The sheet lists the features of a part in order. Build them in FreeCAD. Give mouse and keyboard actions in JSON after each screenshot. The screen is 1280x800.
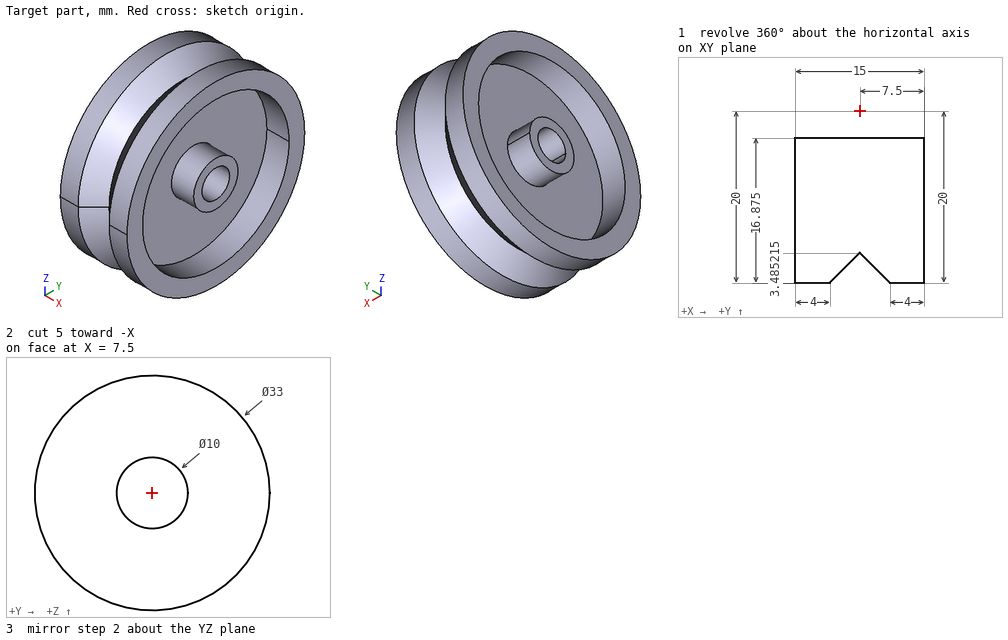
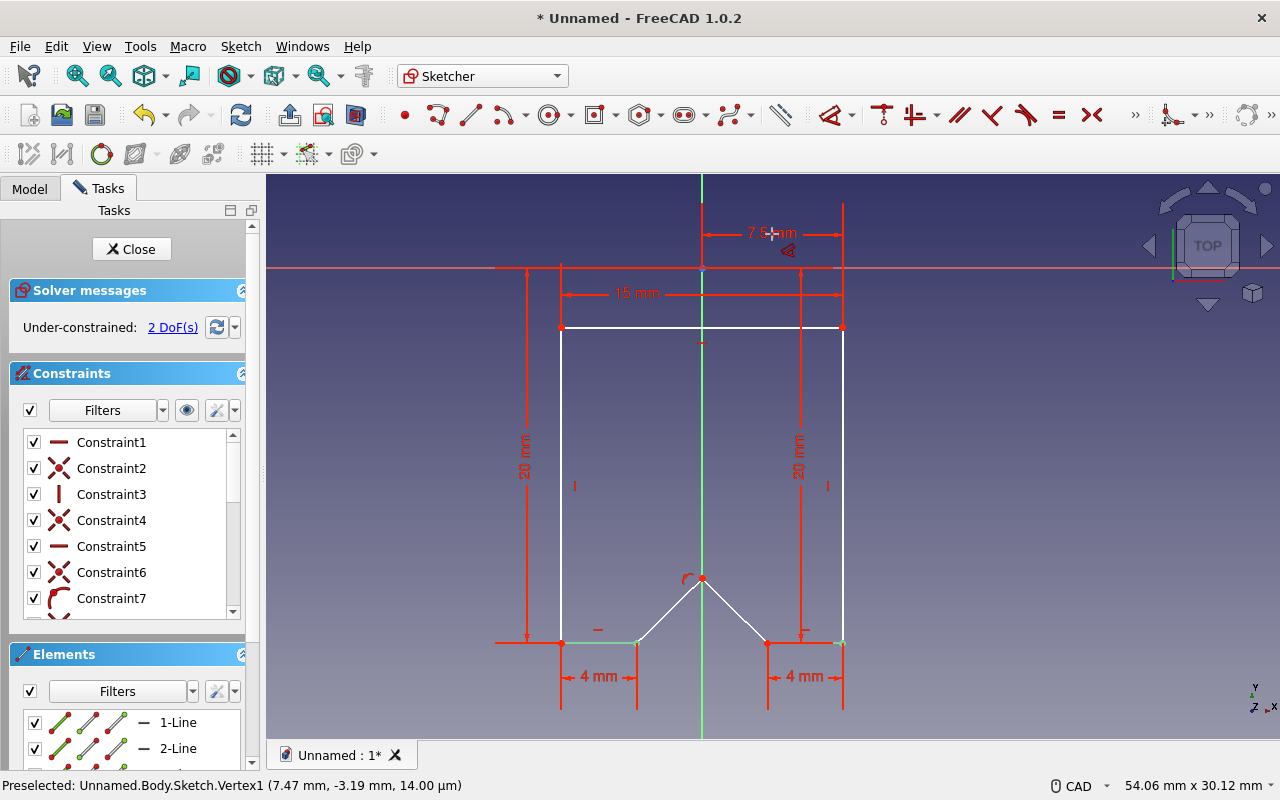
{"action": "left_click", "coordinate": [561, 423]}
{"action": "left_click", "coordinate": [527, 486]}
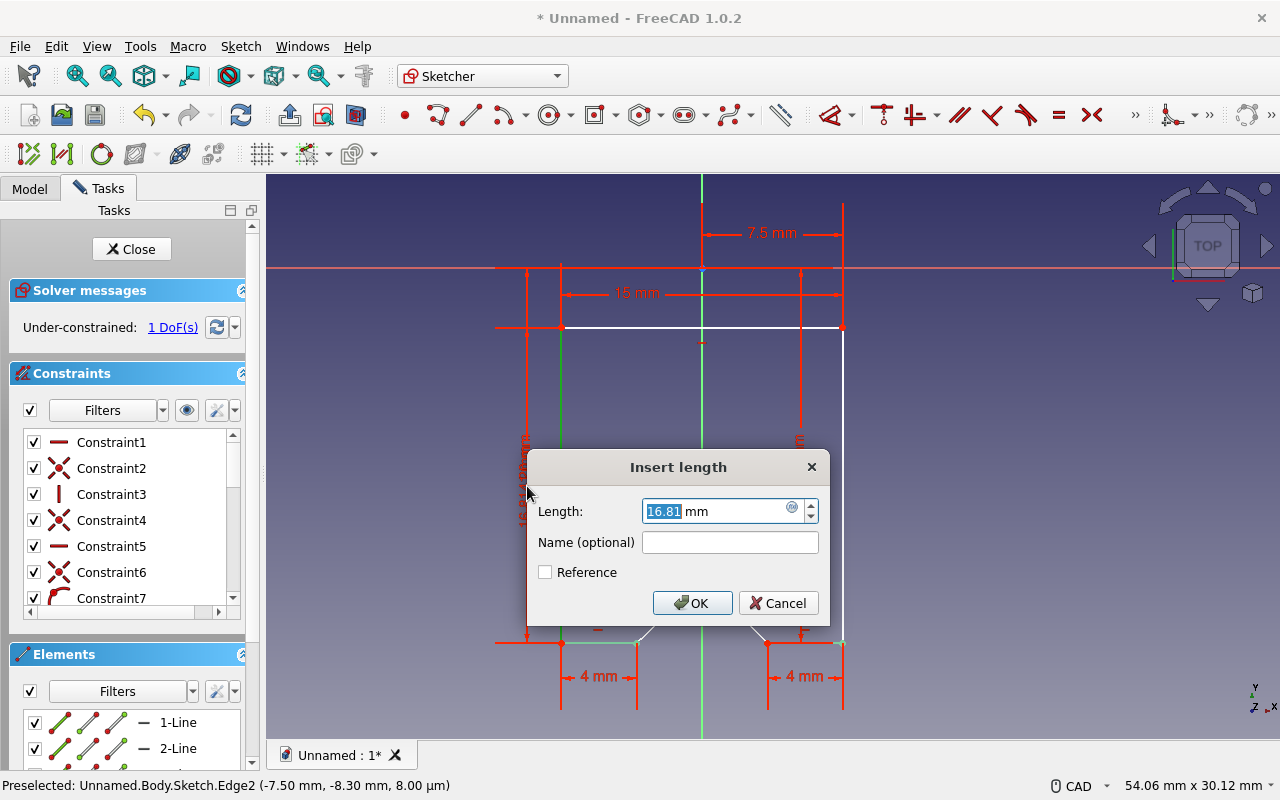
{"action": "type", "text": "16.875"}
{"action": "key", "text": "Return"}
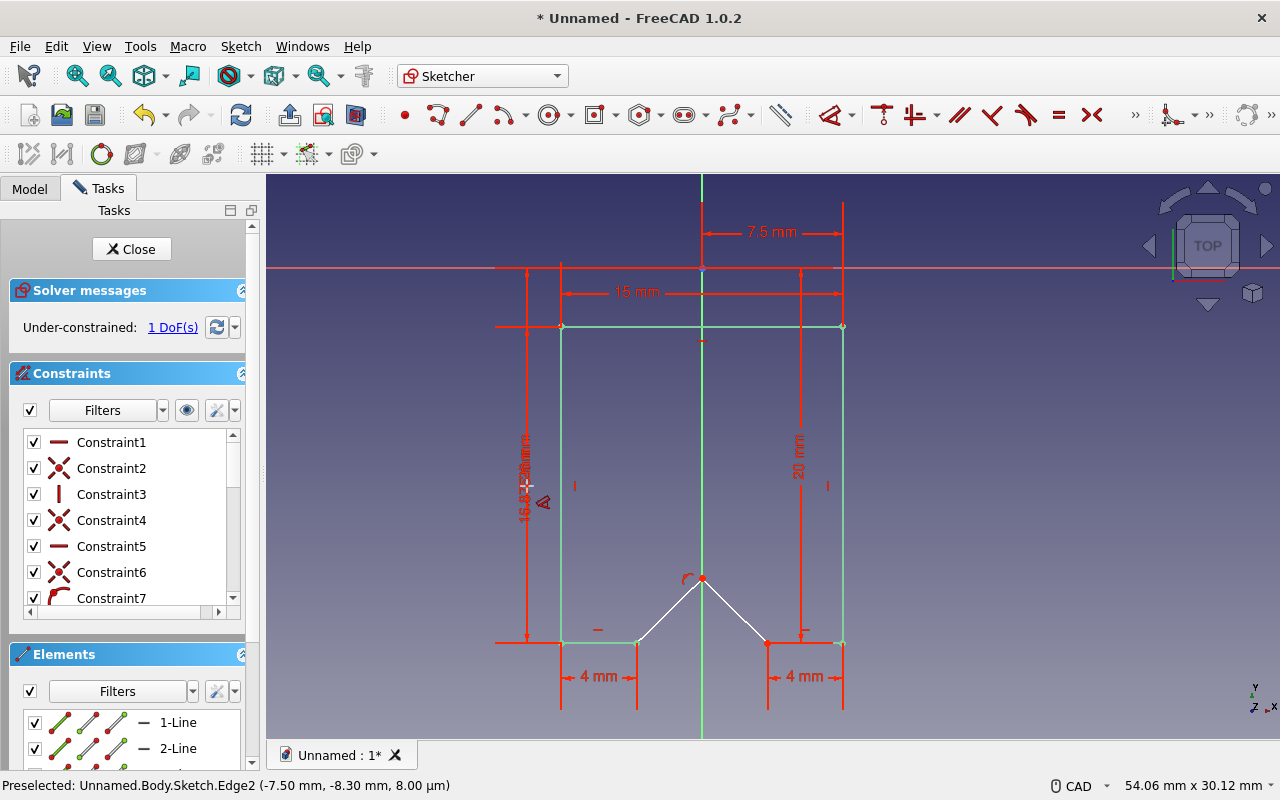
{"action": "left_click", "coordinate": [656, 624]}
{"action": "left_click", "coordinate": [603, 611]}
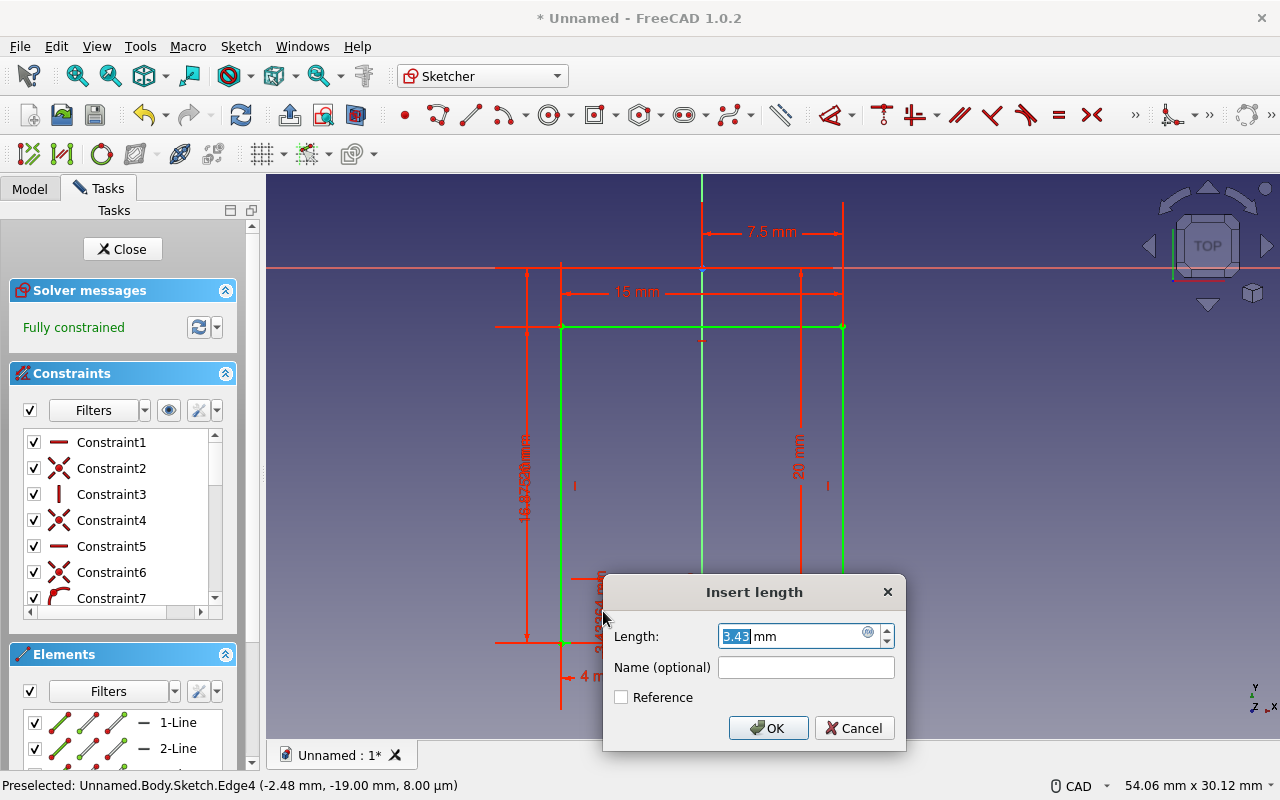
{"action": "type", "text": "3.485215"}
{"action": "key", "text": "Return"}
{"action": "key", "text": "Escape"}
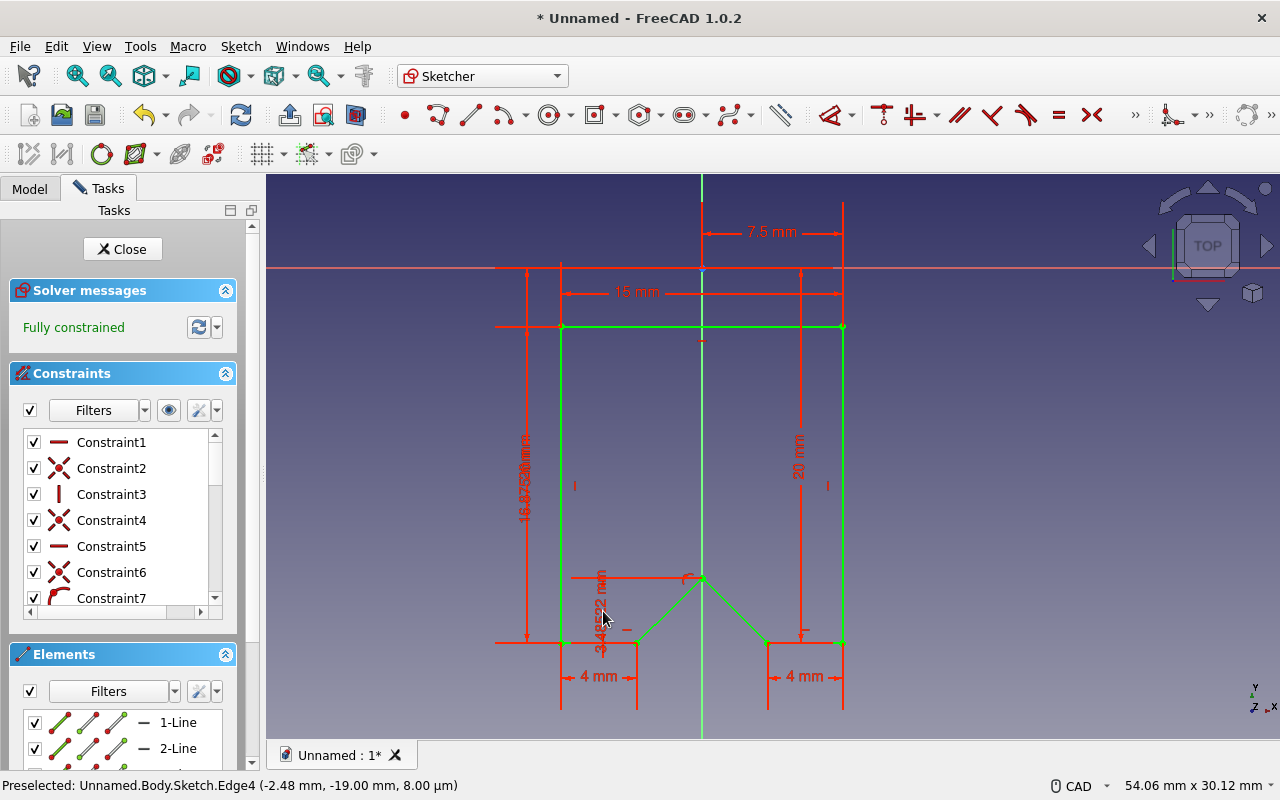
{"action": "left_click", "coordinate": [123, 249]}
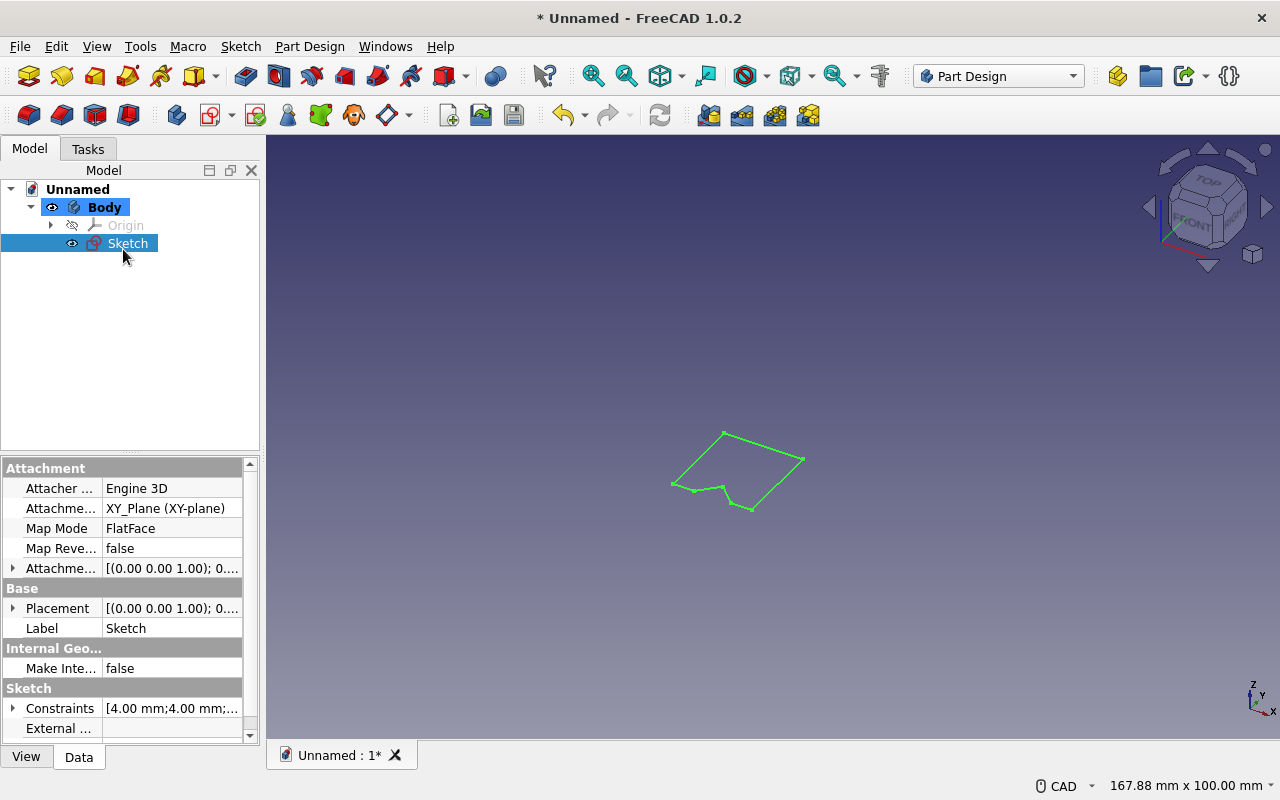
{"action": "left_click", "coordinate": [62, 76]}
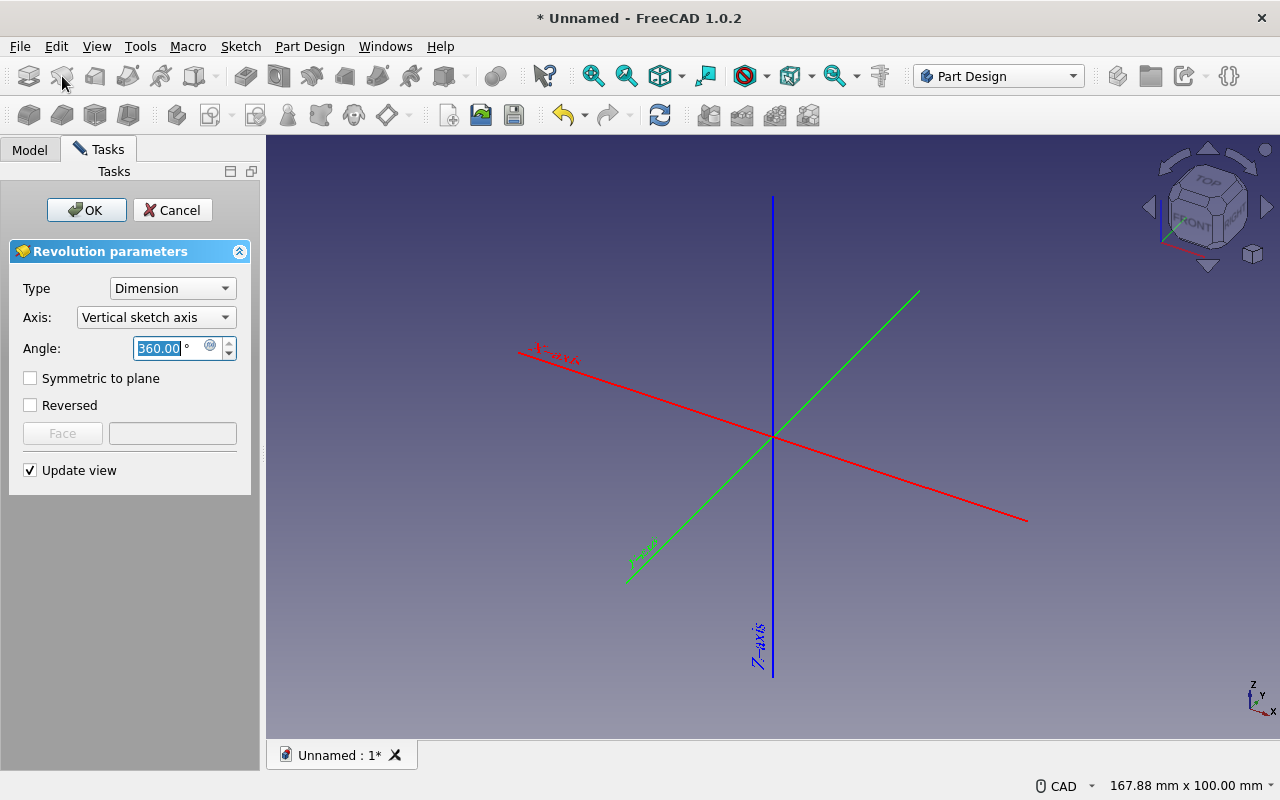
{"action": "left_click", "coordinate": [157, 318]}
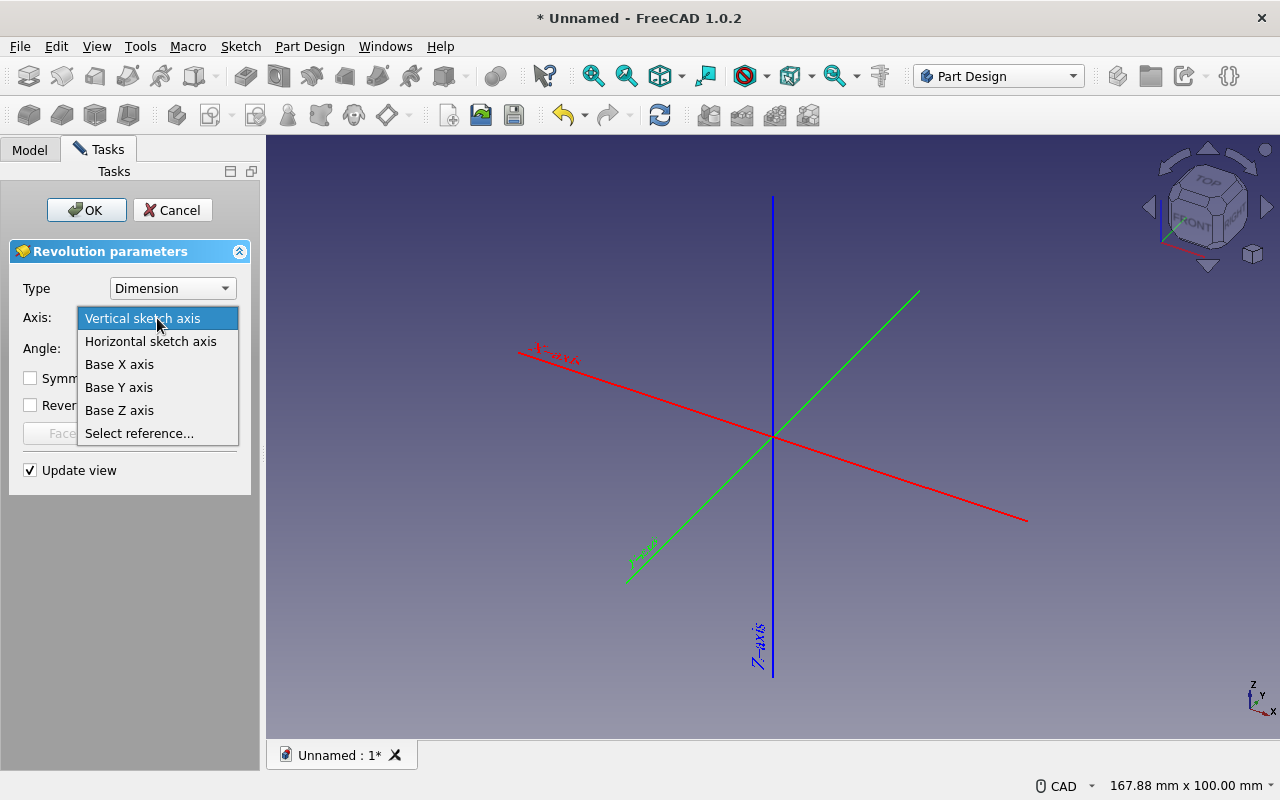
{"action": "left_click", "coordinate": [156, 342]}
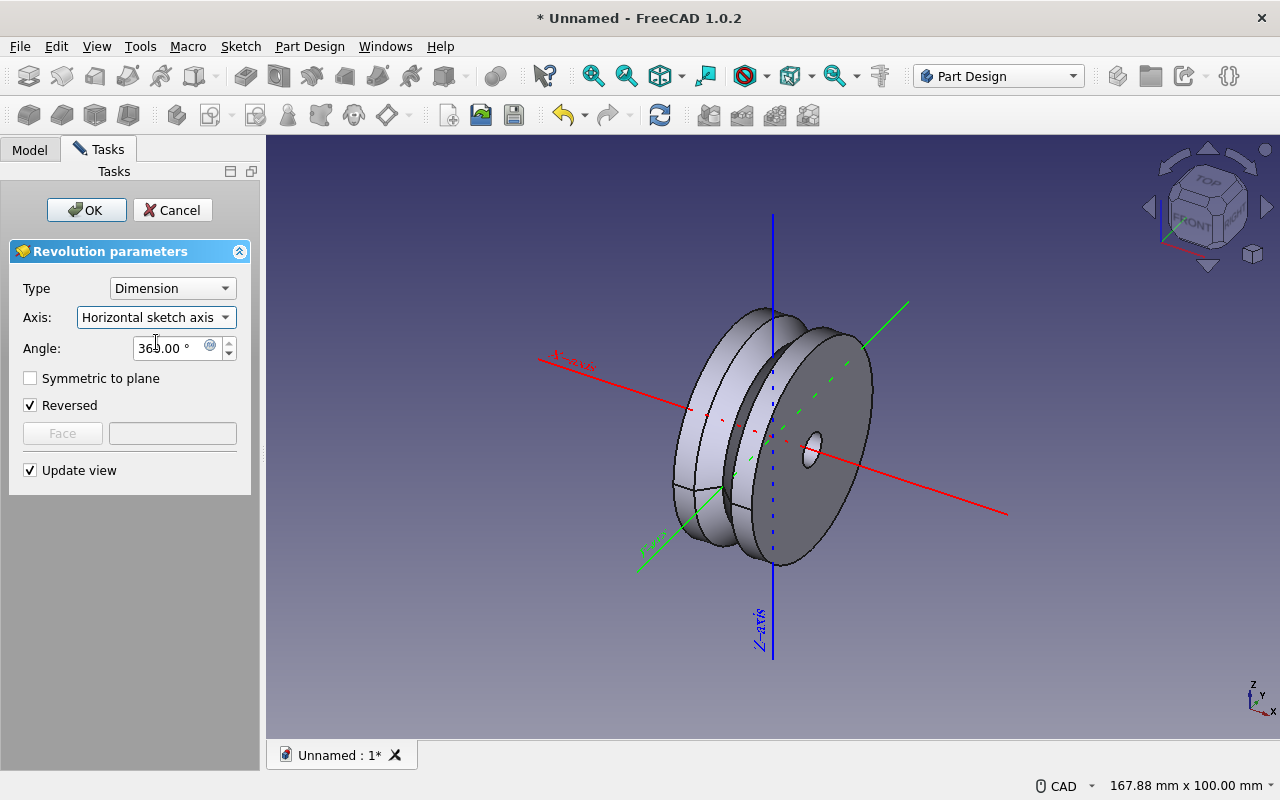
{"action": "left_click", "coordinate": [87, 210]}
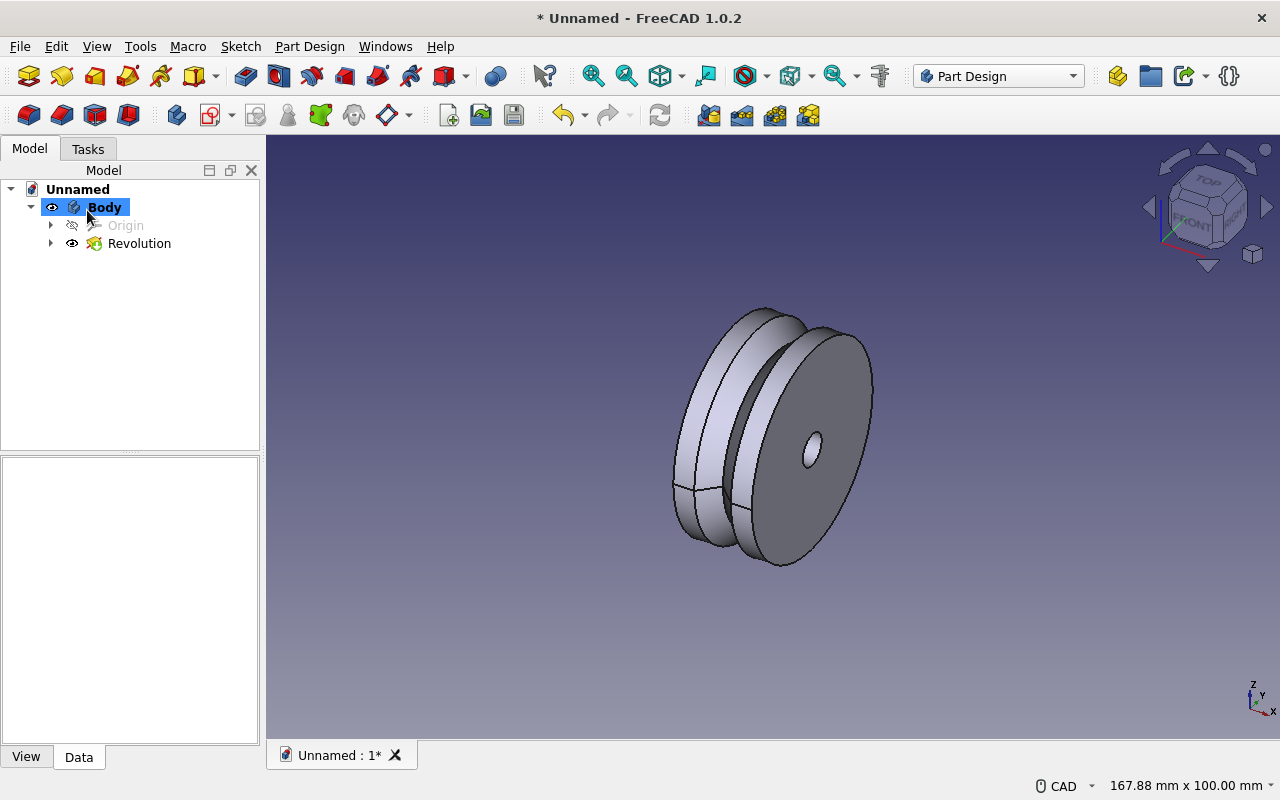
{"action": "left_click", "coordinate": [847, 415]}